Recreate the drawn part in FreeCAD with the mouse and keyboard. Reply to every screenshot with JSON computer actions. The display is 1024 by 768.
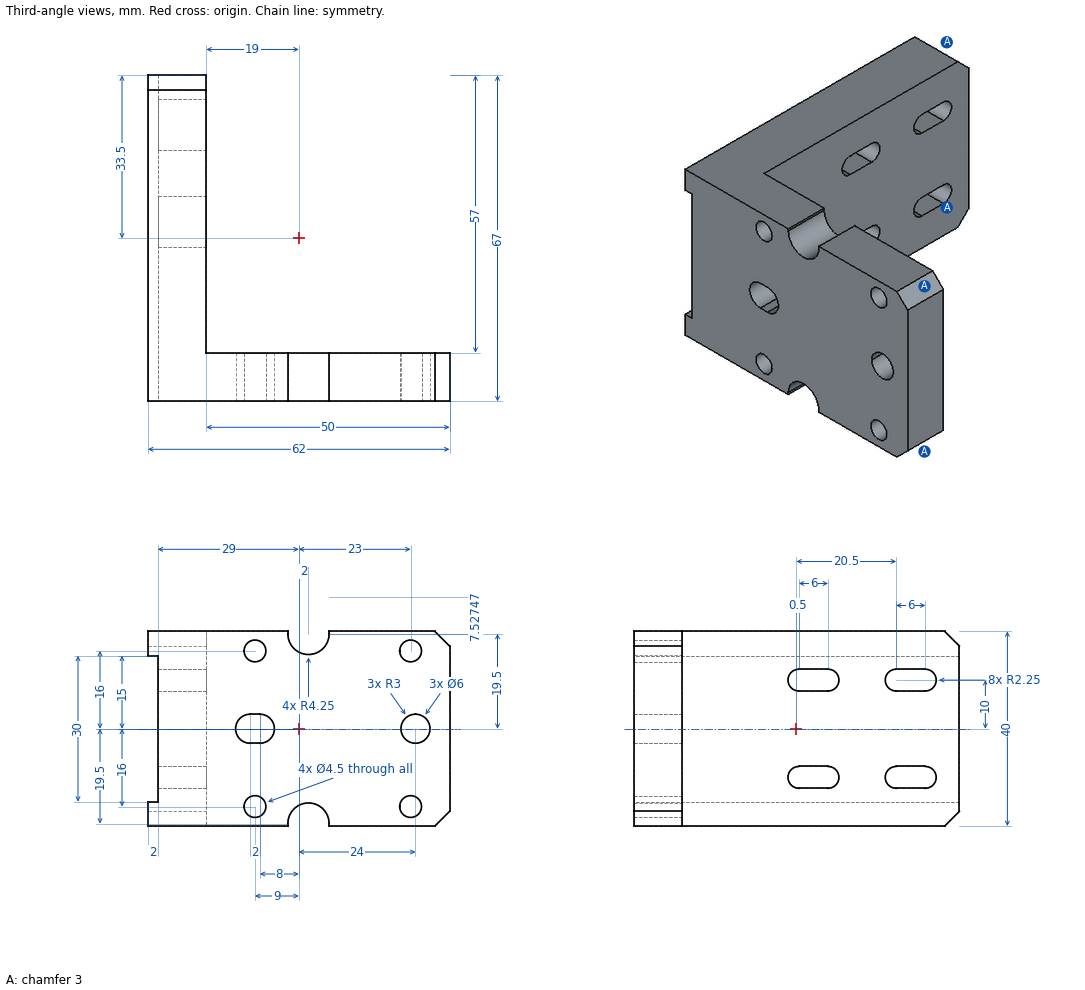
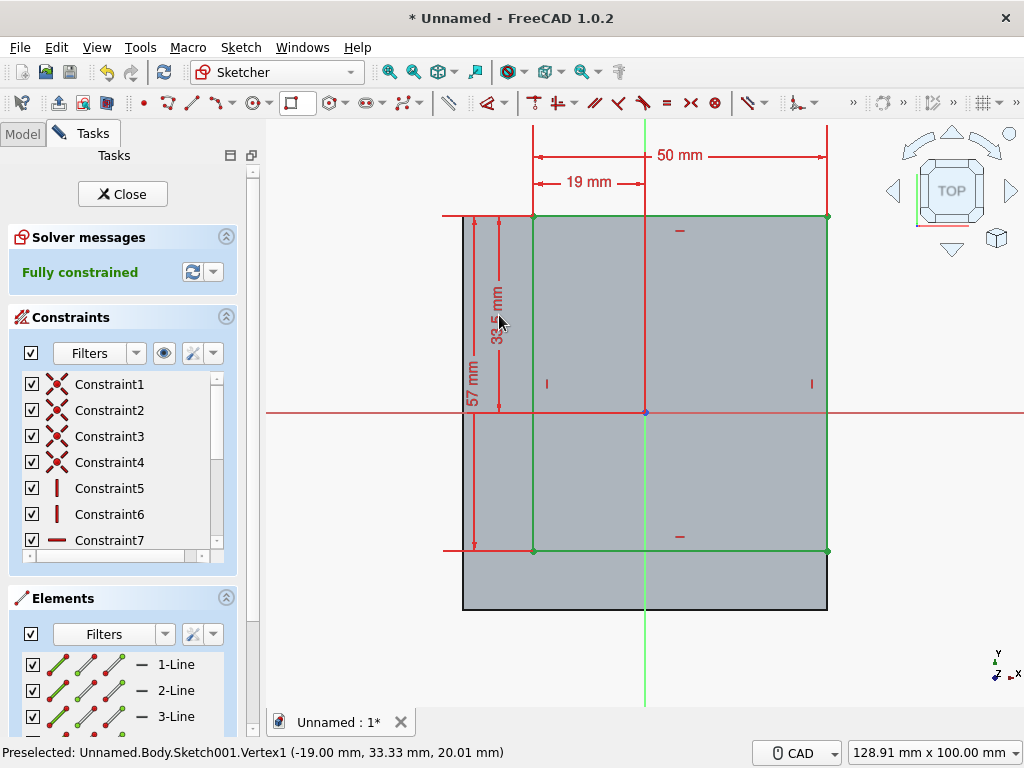
{"action": "left_click", "coordinate": [123, 194]}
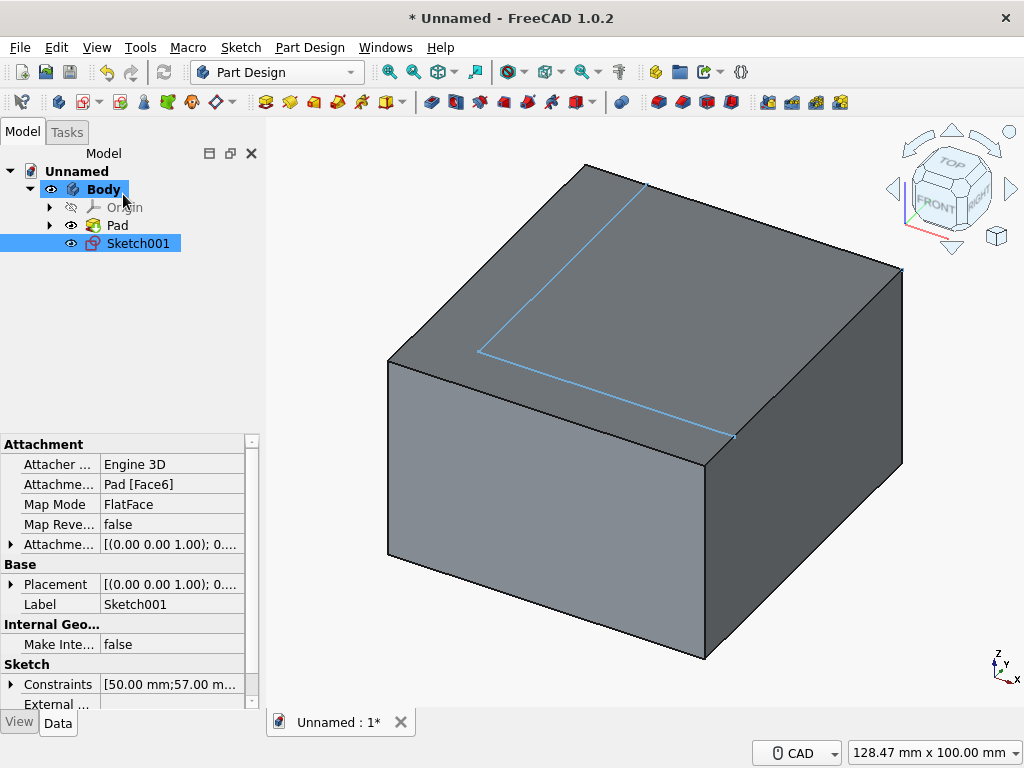
{"action": "left_click", "coordinate": [432, 102]}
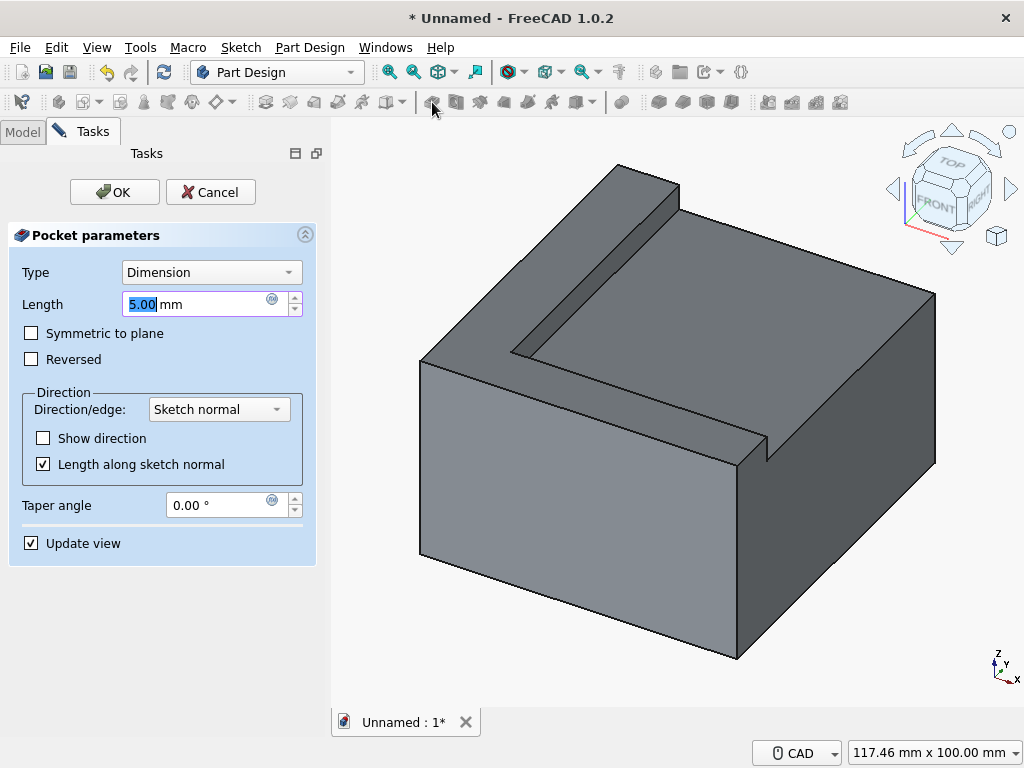
{"action": "left_click", "coordinate": [212, 272]}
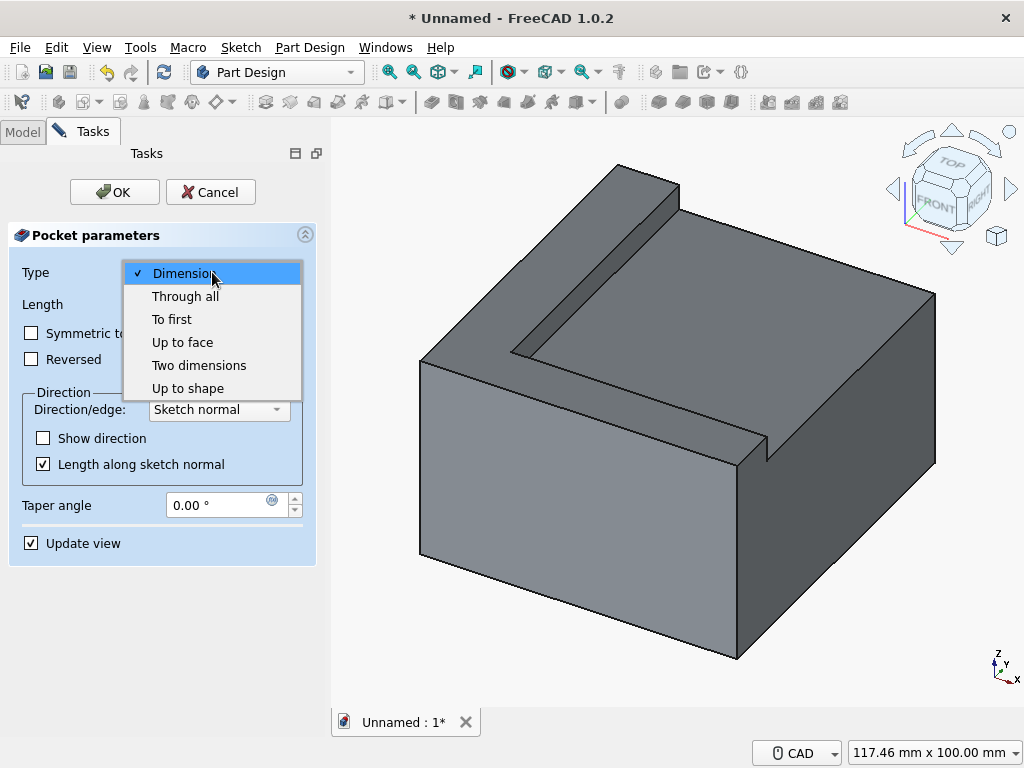
{"action": "left_click", "coordinate": [212, 296]}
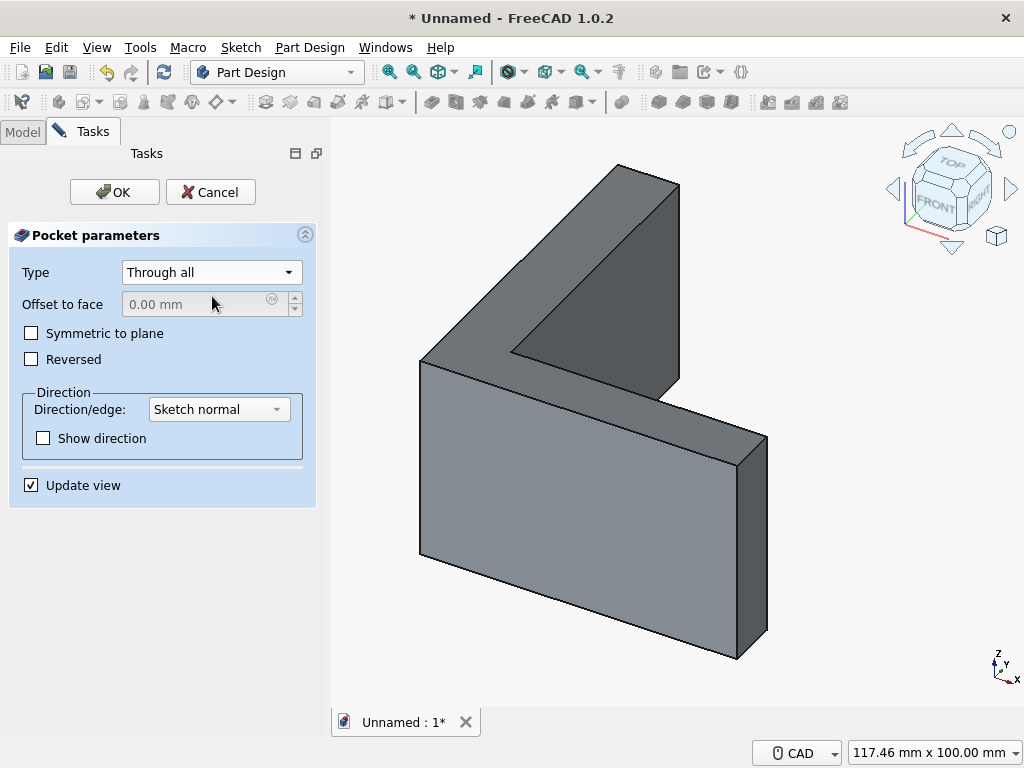
{"action": "left_click", "coordinate": [115, 192]}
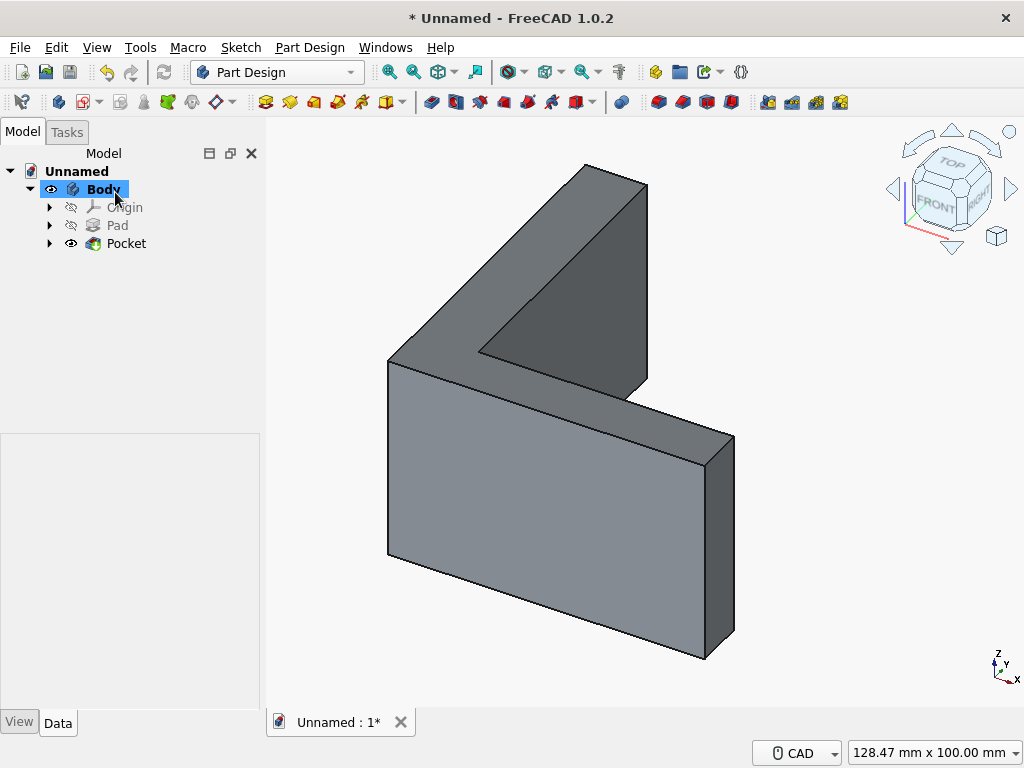
{"action": "key", "text": "4"}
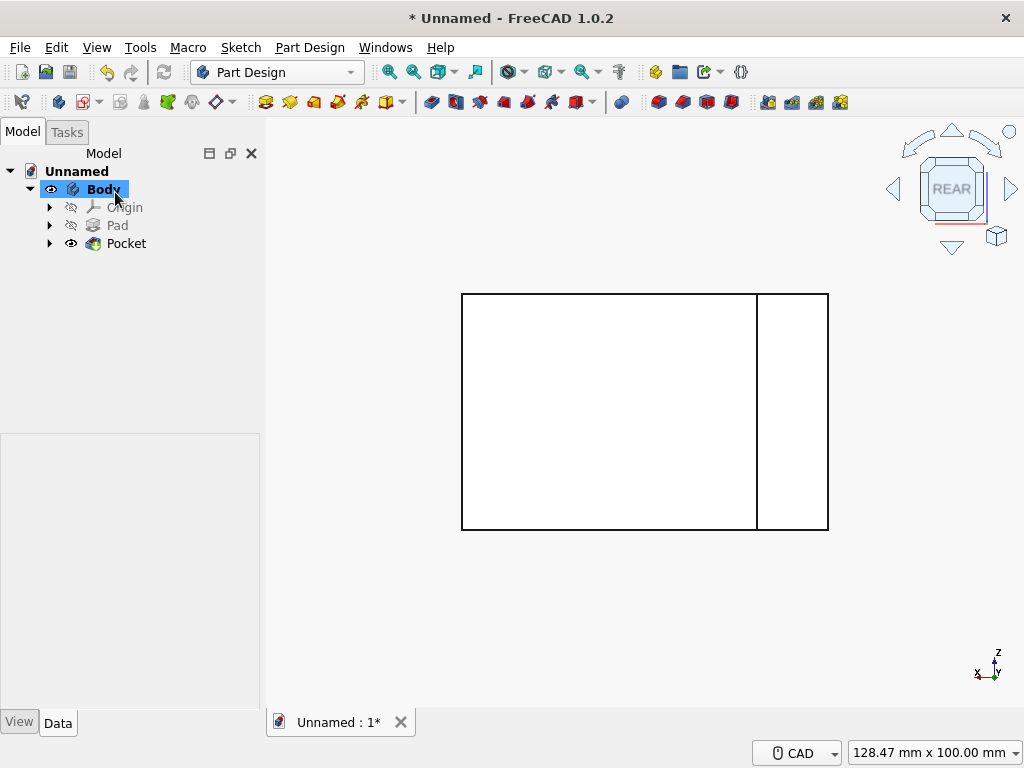
{"action": "left_click", "coordinate": [793, 344]}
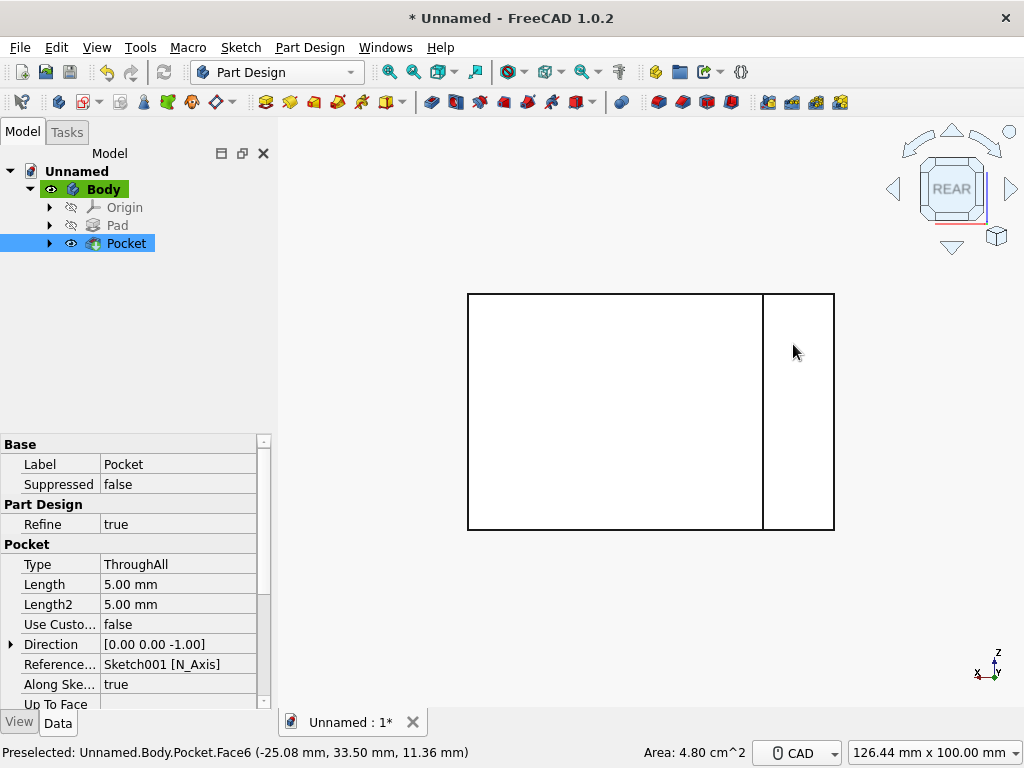
{"action": "left_click", "coordinate": [84, 102]}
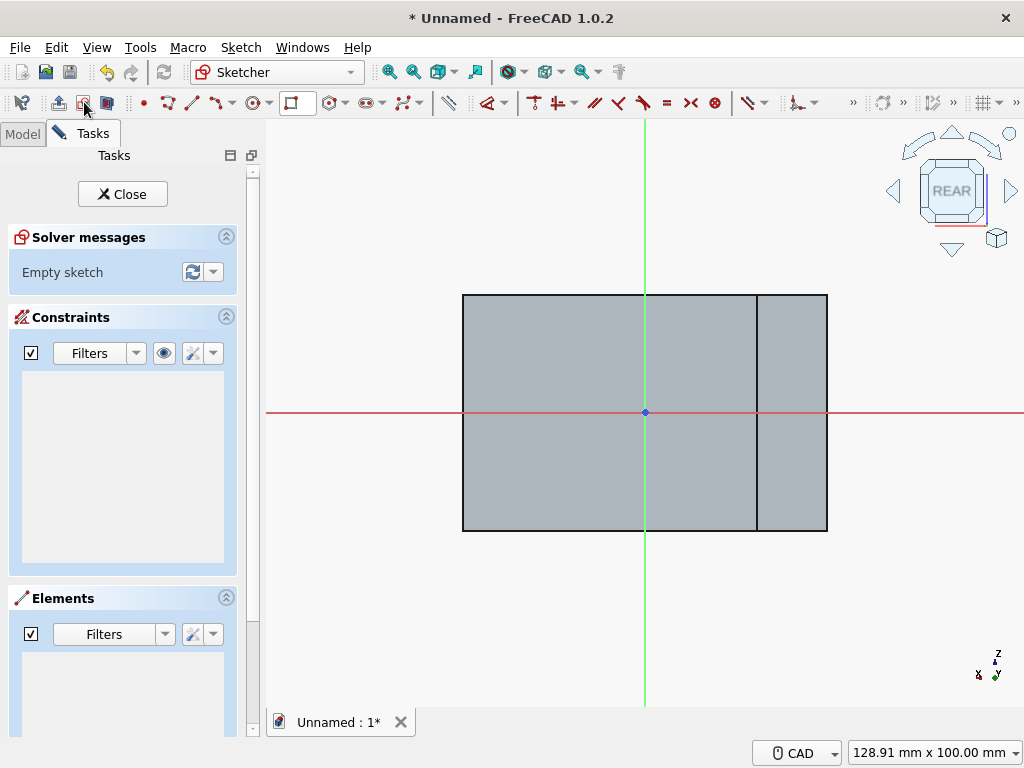
{"action": "scroll", "coordinate": [859, 413], "scroll_direction": "up", "scroll_amount": 4}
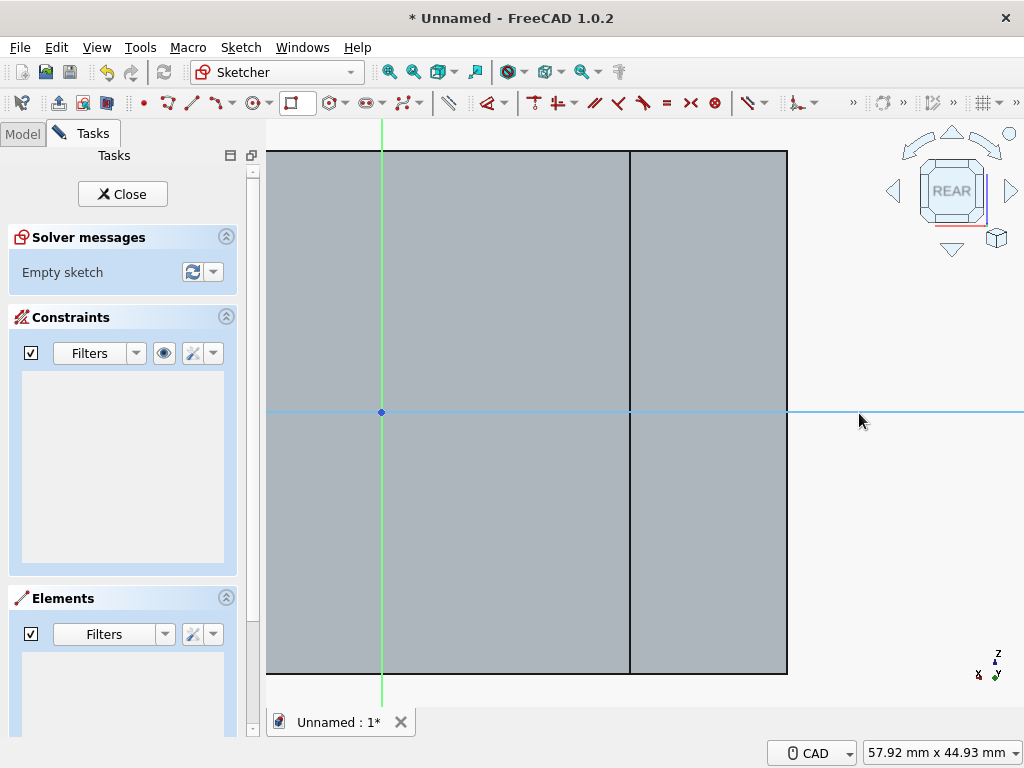
{"action": "left_click", "coordinate": [292, 104]}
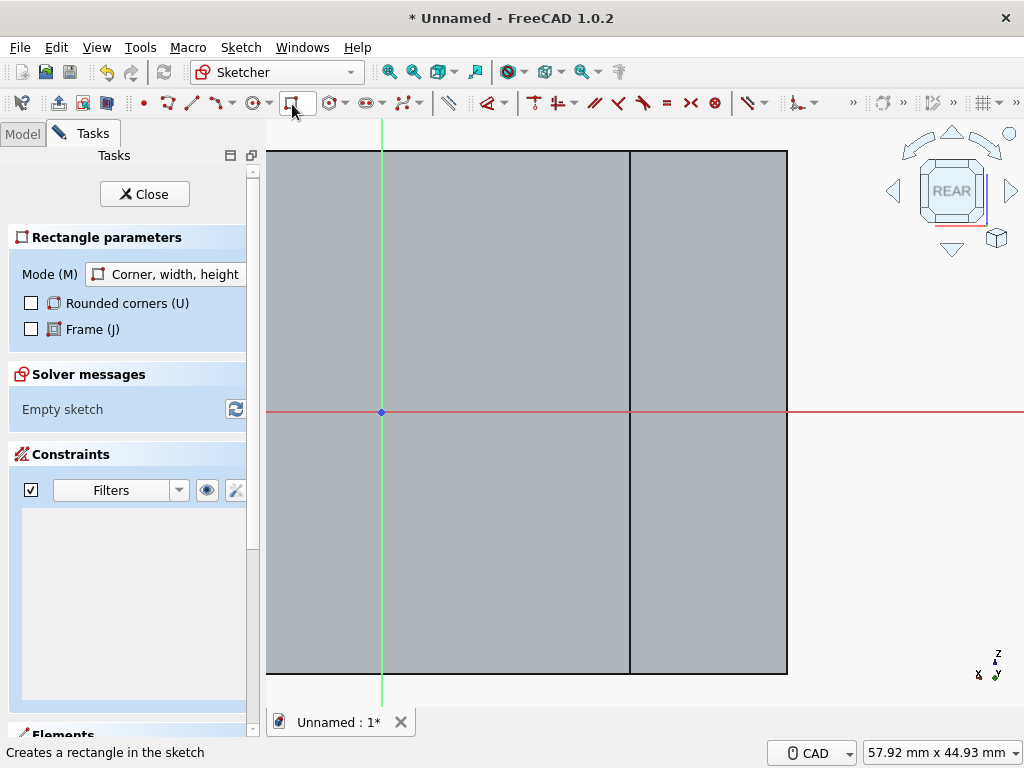
{"action": "left_click", "coordinate": [761, 216]}
{"action": "mouse_move", "coordinate": [787, 609]}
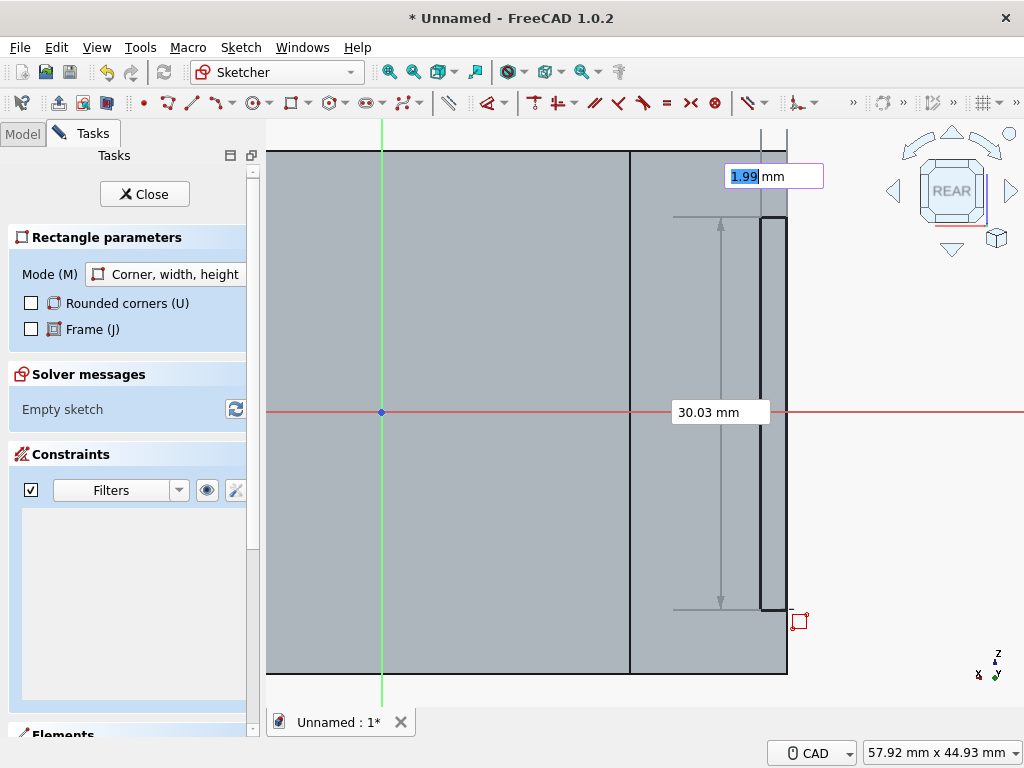
{"action": "type", "text": "2"}
{"action": "key", "text": "Tab"}
{"action": "type", "text": "30"}
{"action": "key", "text": "Return"}
{"action": "key", "text": "Escape"}